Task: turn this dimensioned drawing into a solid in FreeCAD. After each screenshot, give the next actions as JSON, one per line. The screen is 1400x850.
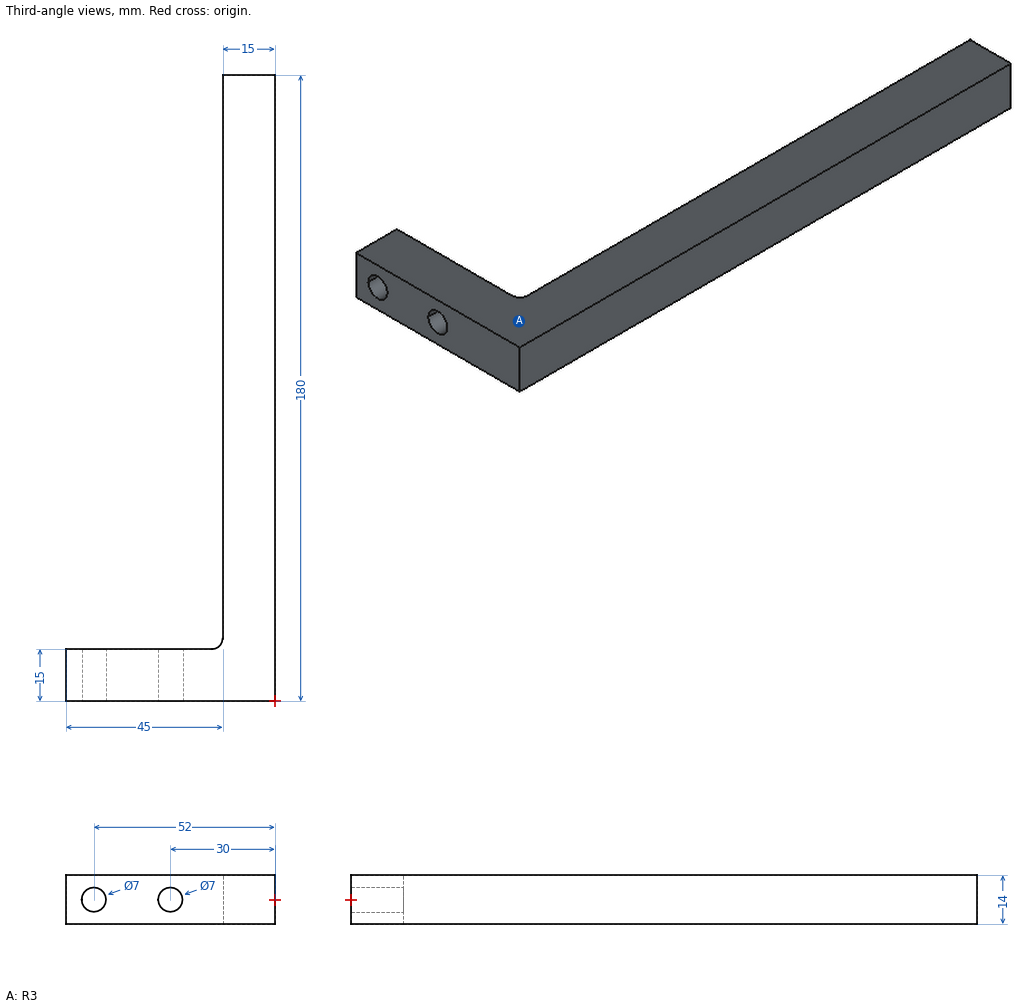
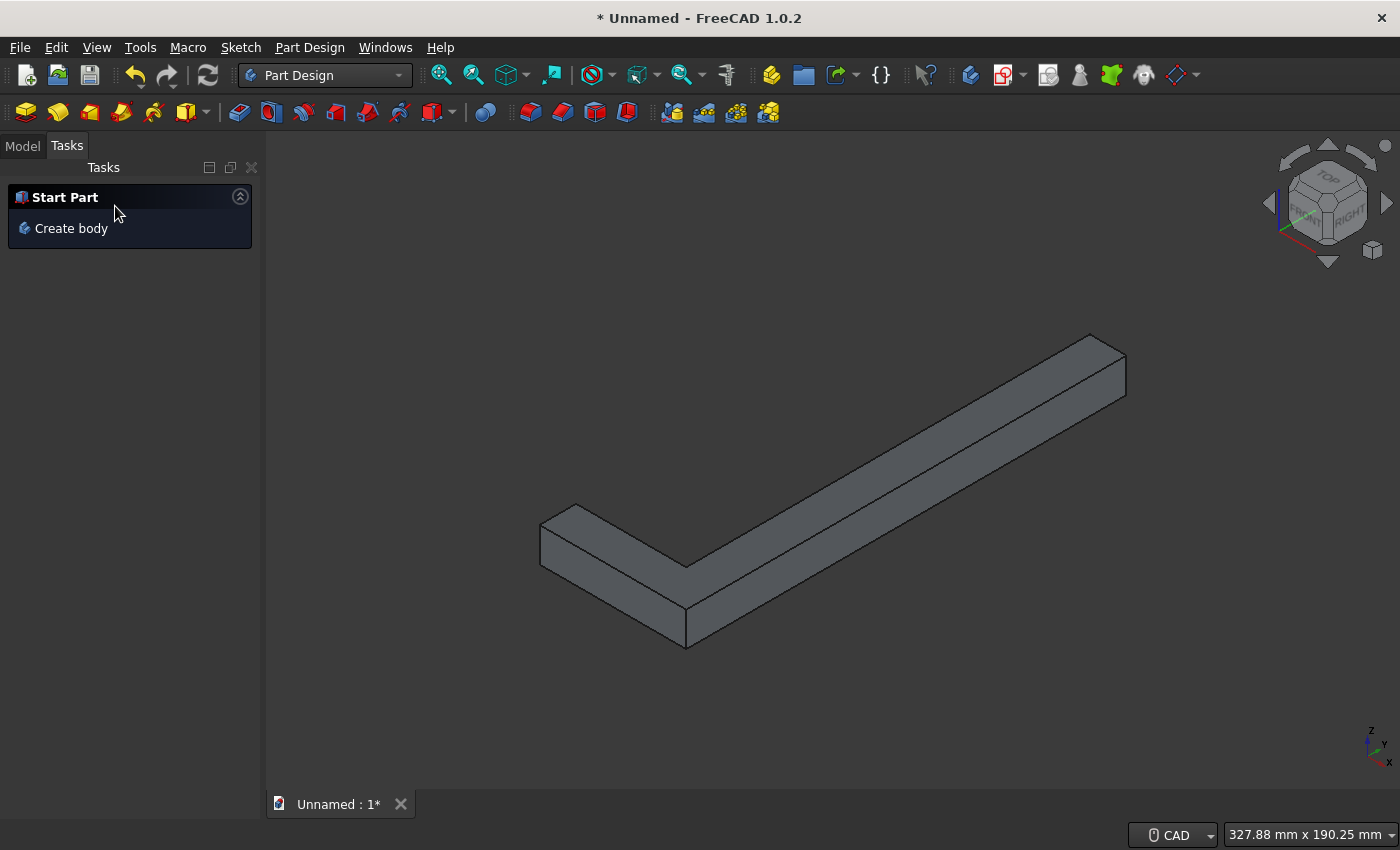
{"action": "key", "text": "2"}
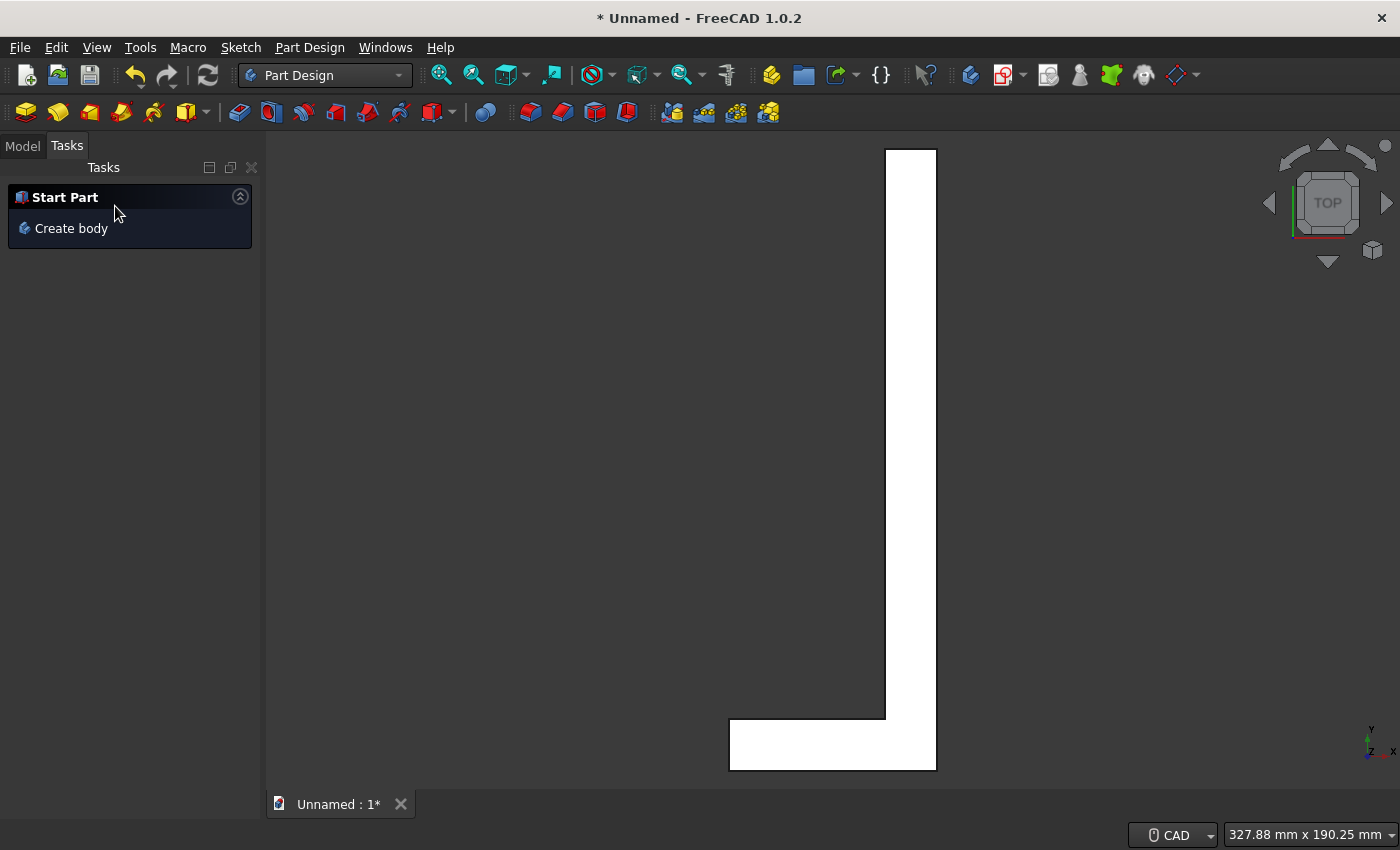
{"action": "key", "text": "1"}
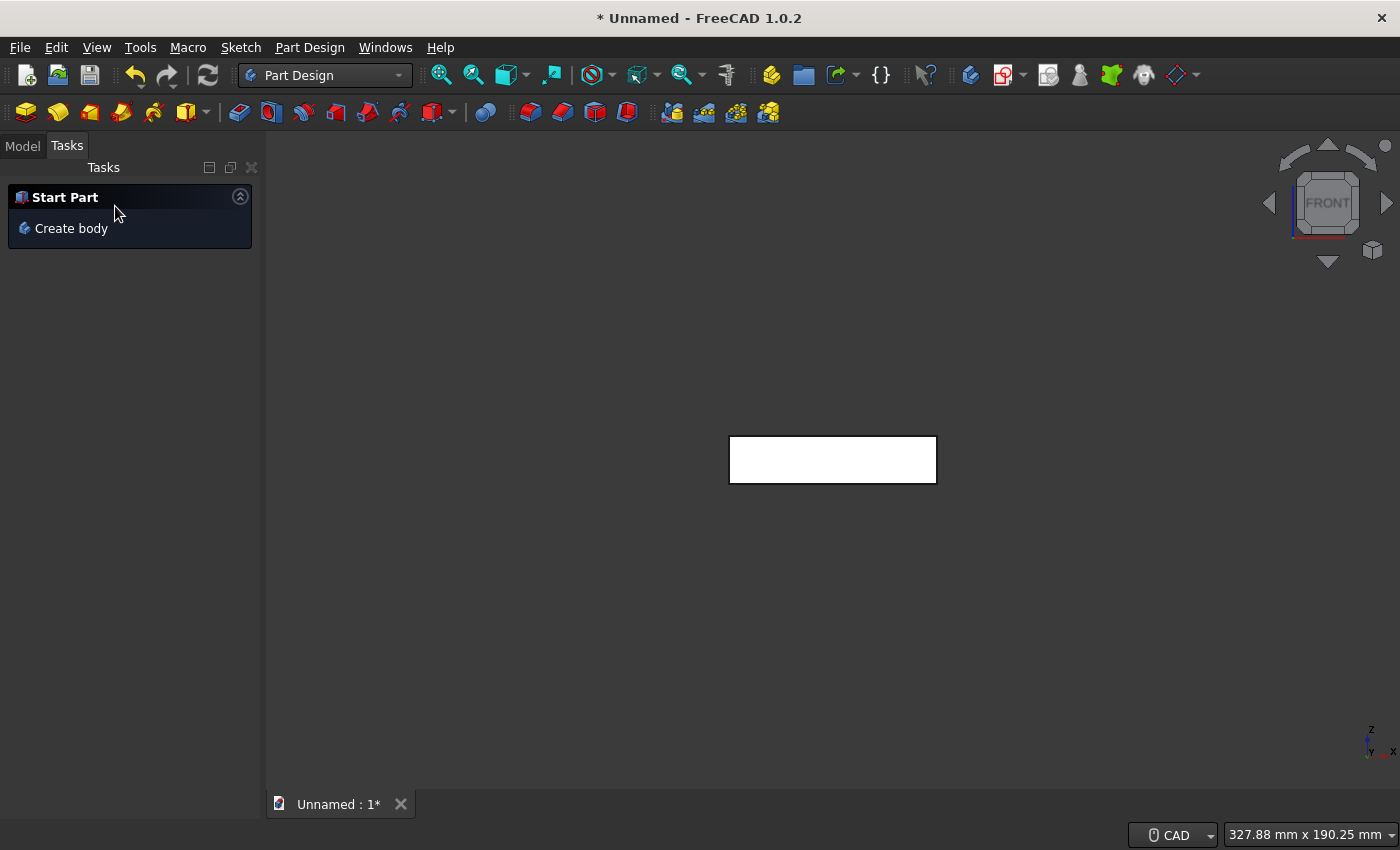
{"action": "key", "text": "v f"}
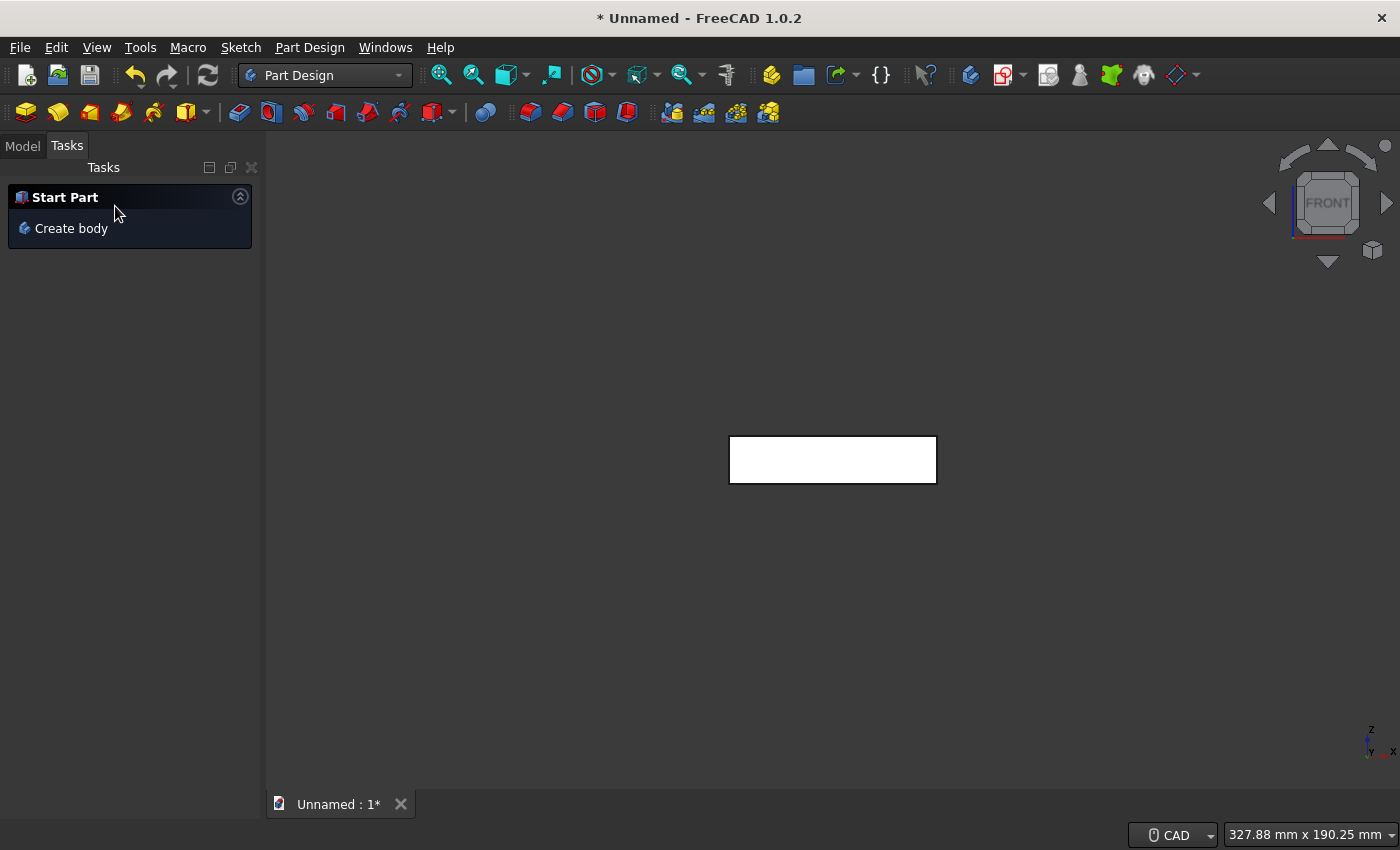
{"action": "key", "text": "3"}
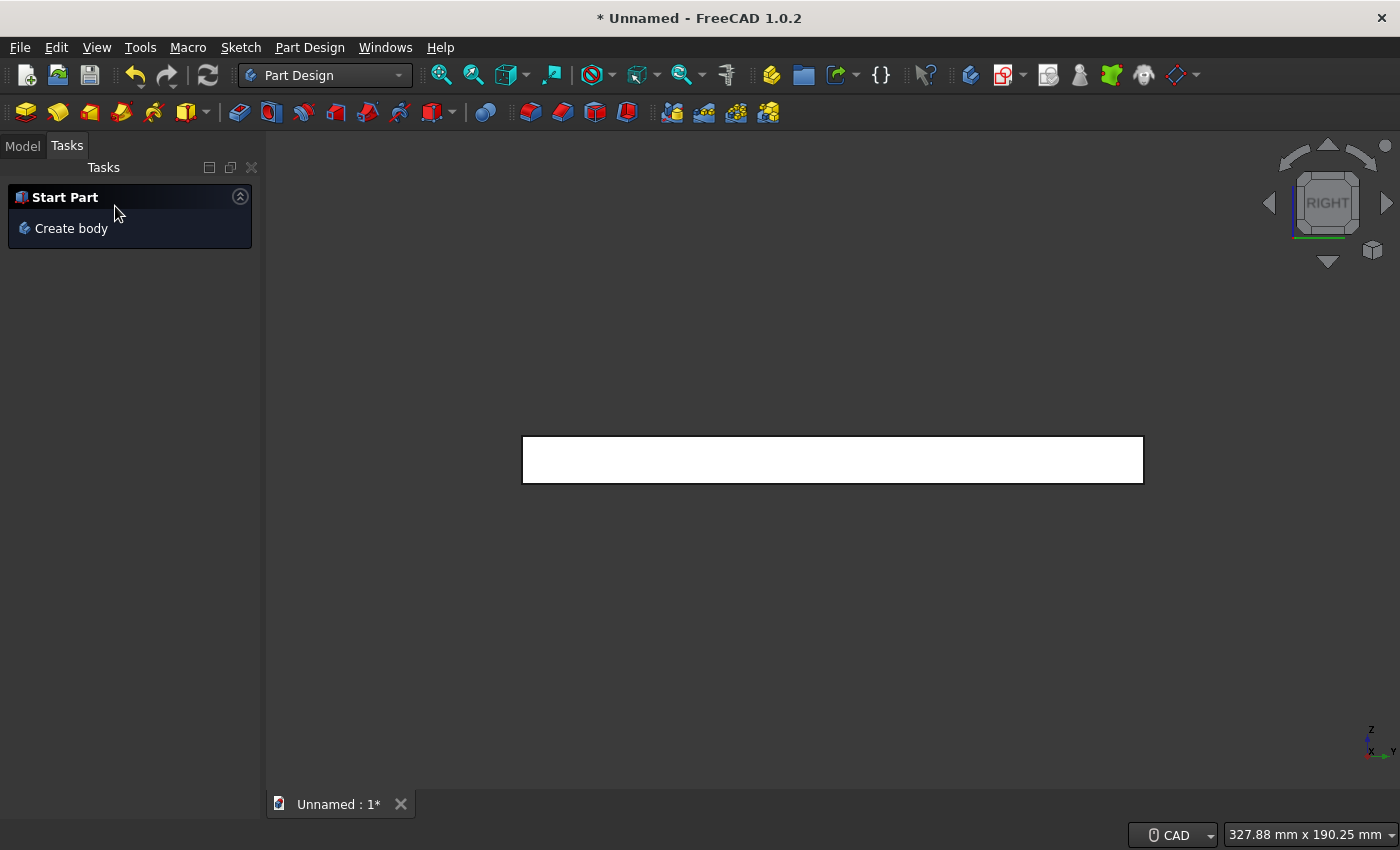
{"action": "key", "text": "5"}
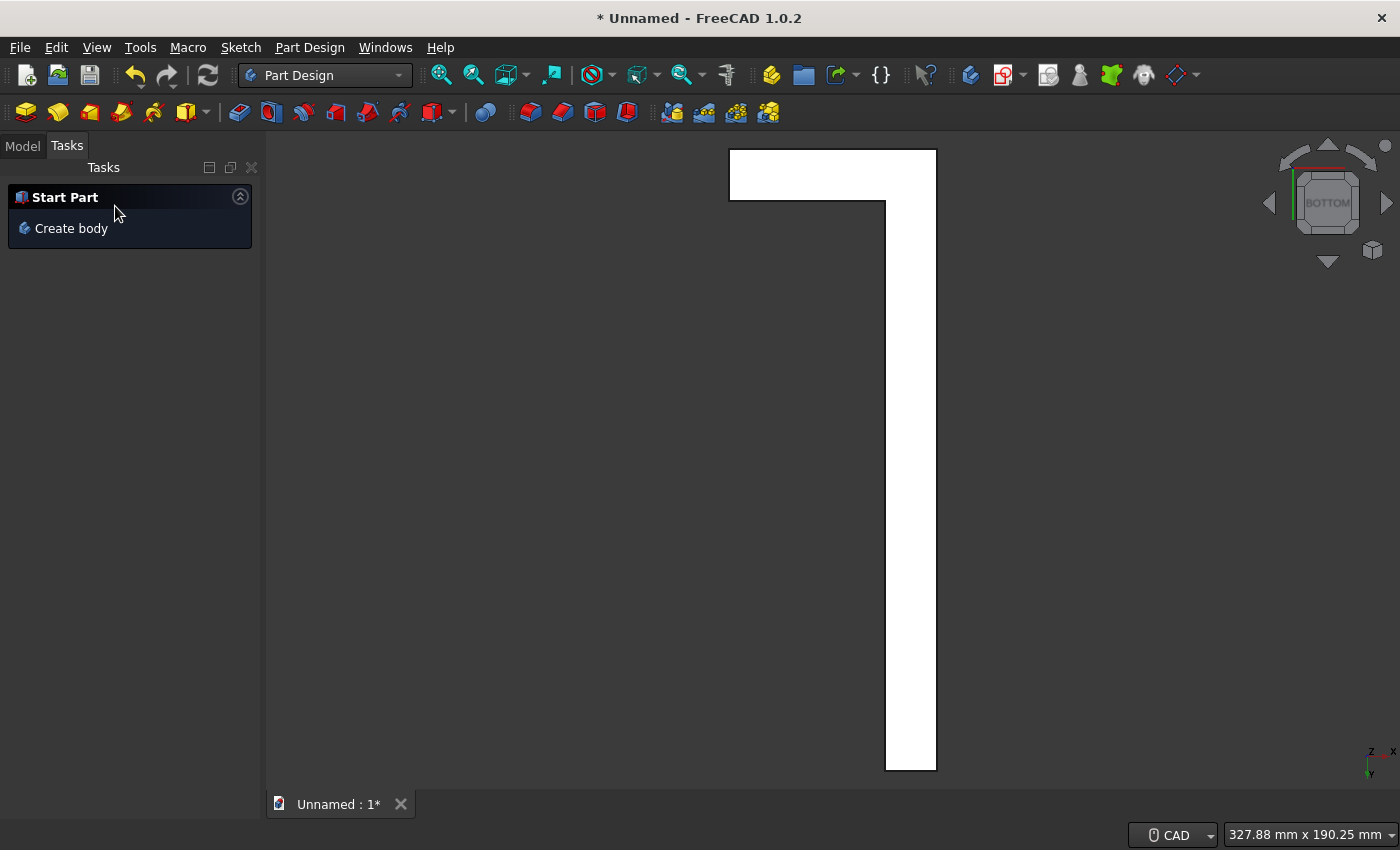
{"action": "key", "text": "4"}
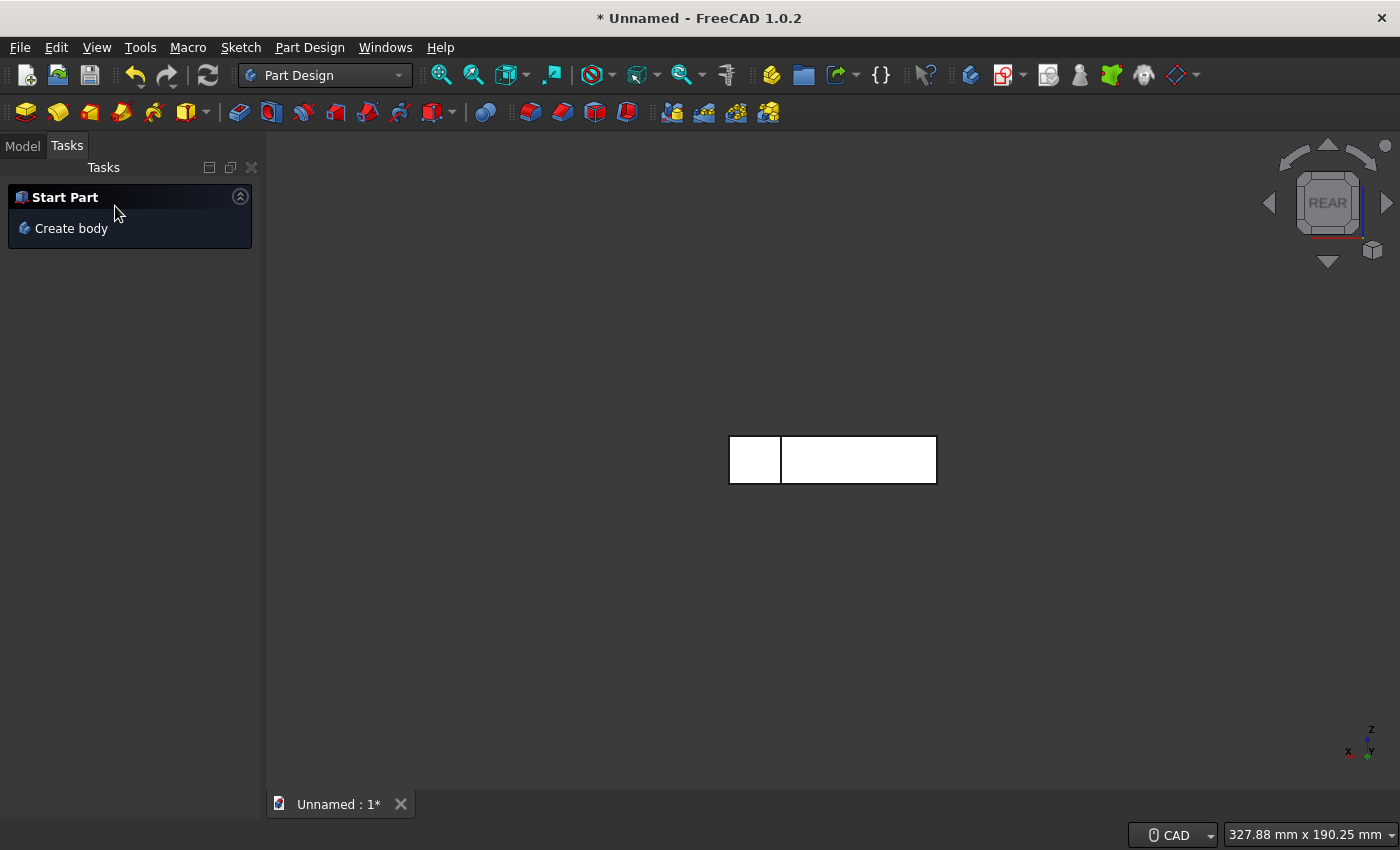
{"action": "left_click", "coordinate": [442, 76]}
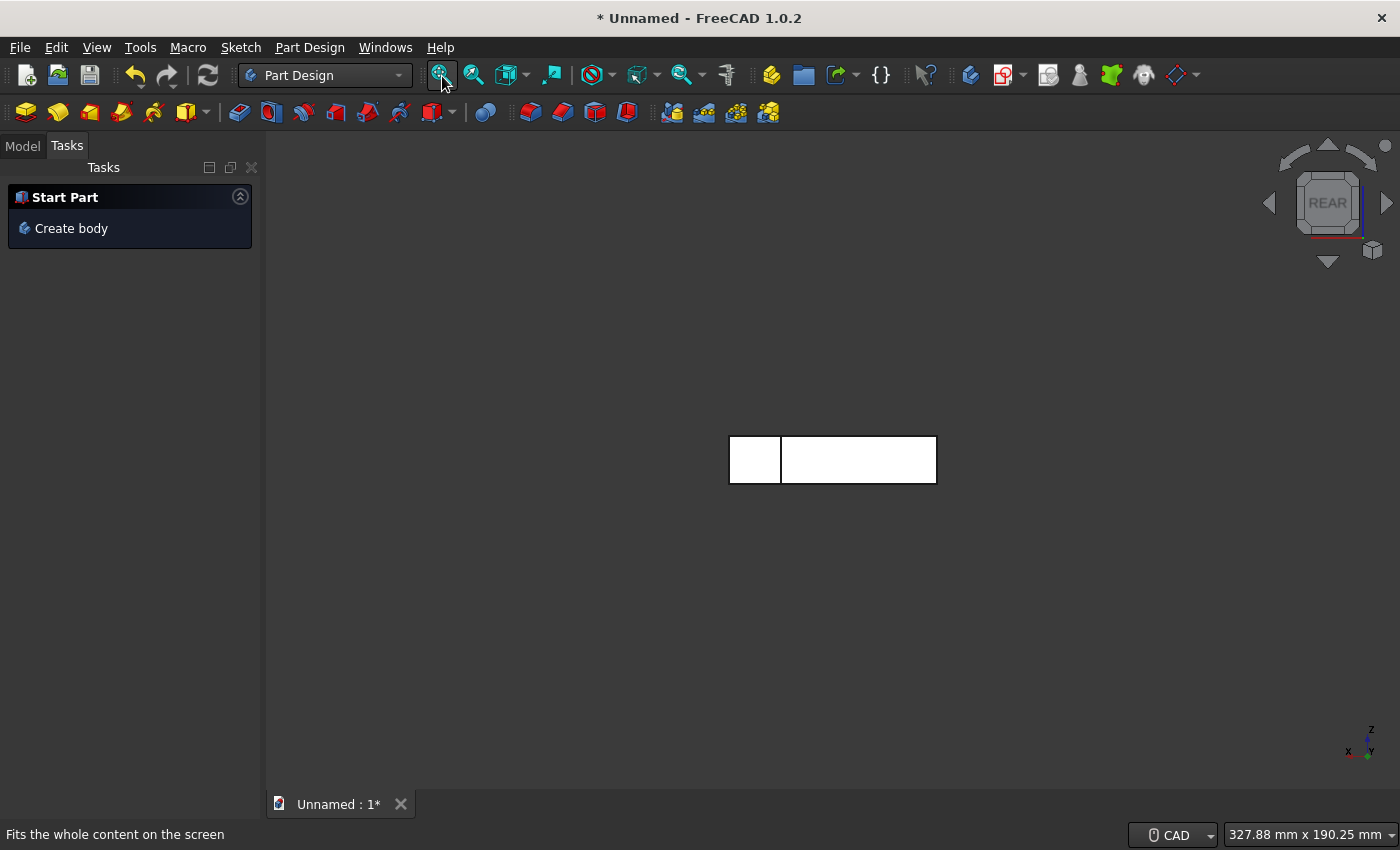
{"action": "key", "text": "6"}